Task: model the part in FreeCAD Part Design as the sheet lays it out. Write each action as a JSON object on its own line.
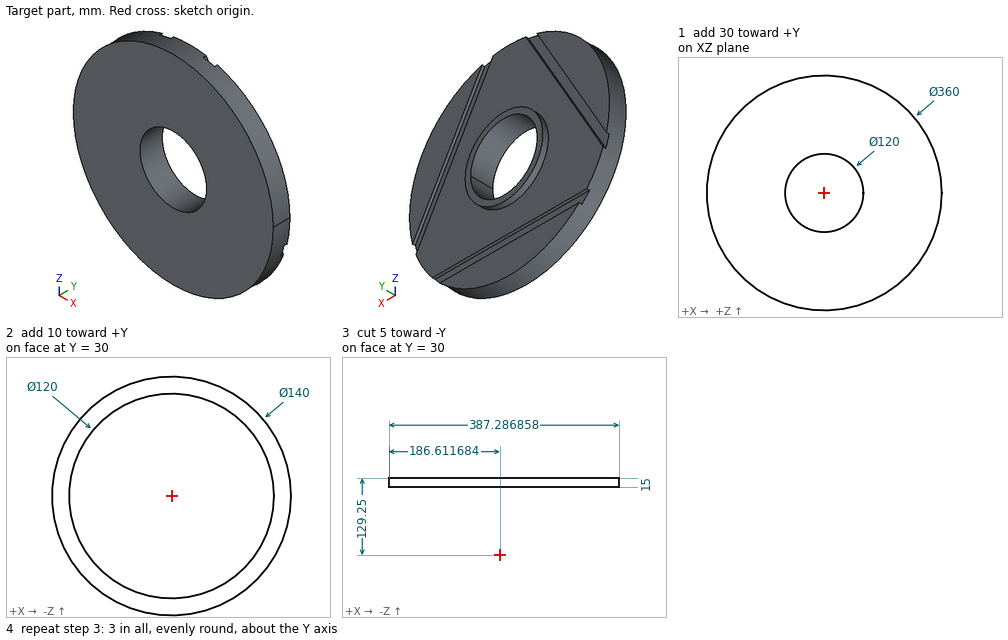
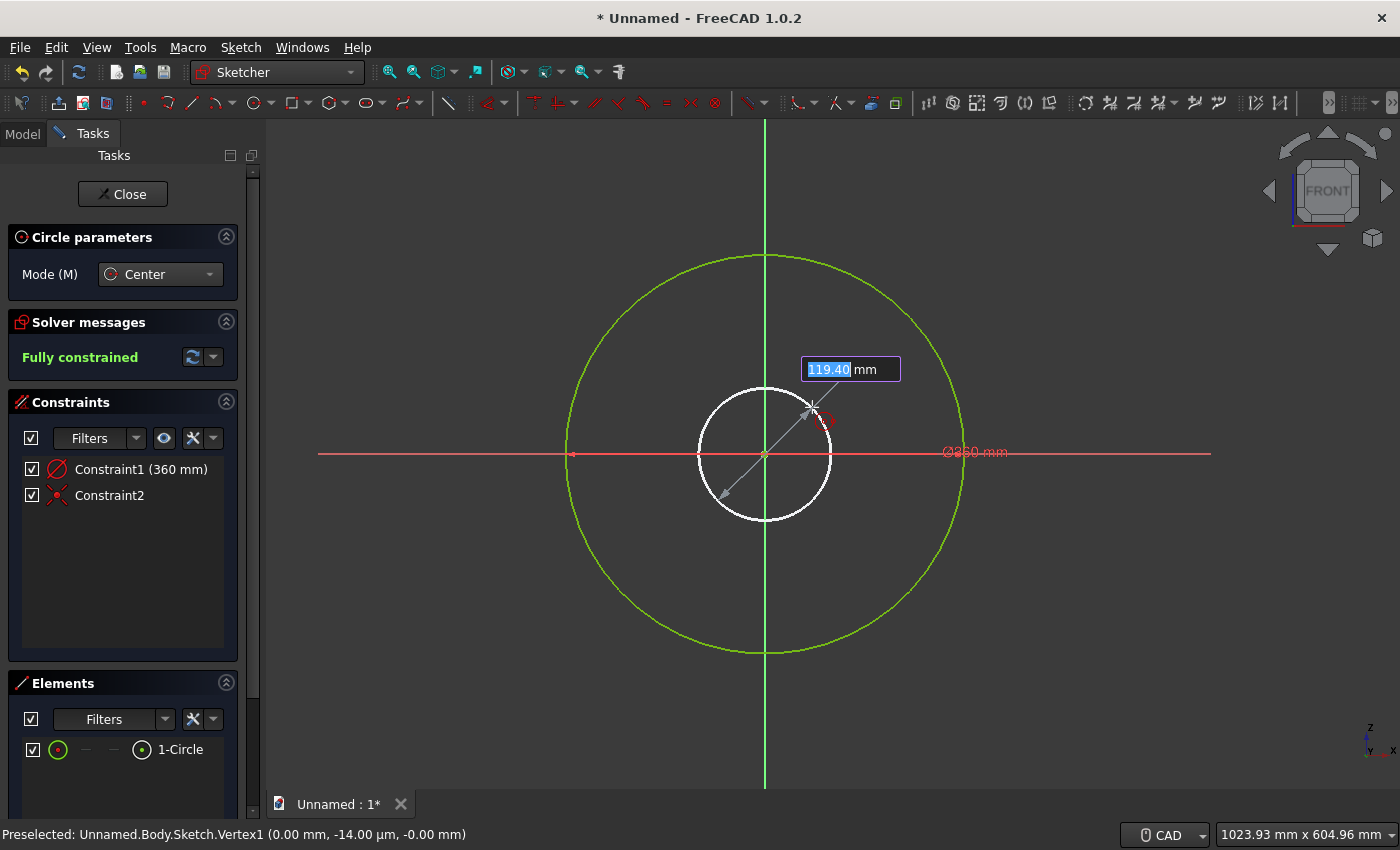
{"action": "type", "text": "120"}
{"action": "key", "text": "Return"}
{"action": "key", "text": "Escape"}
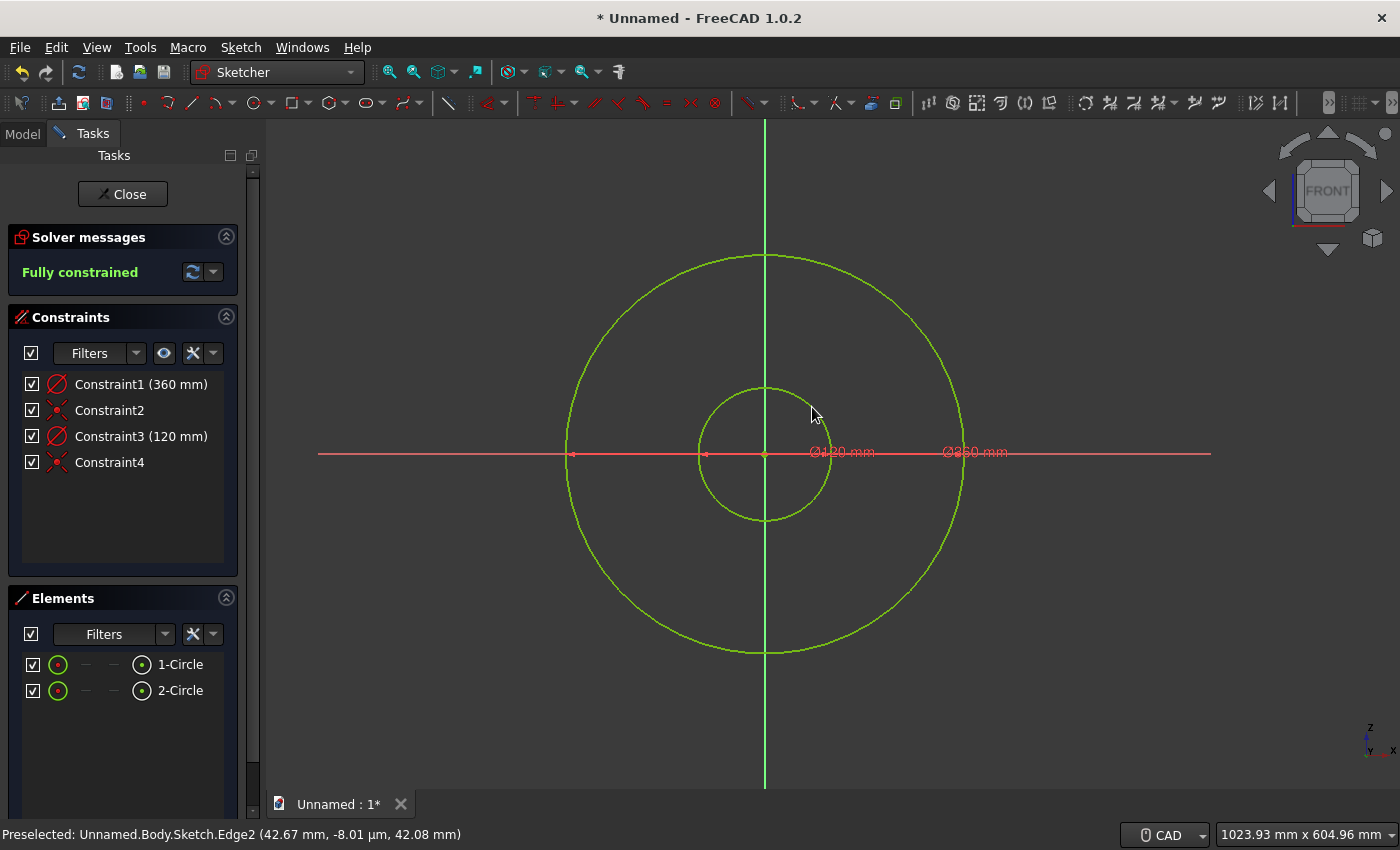
{"action": "left_click", "coordinate": [123, 194]}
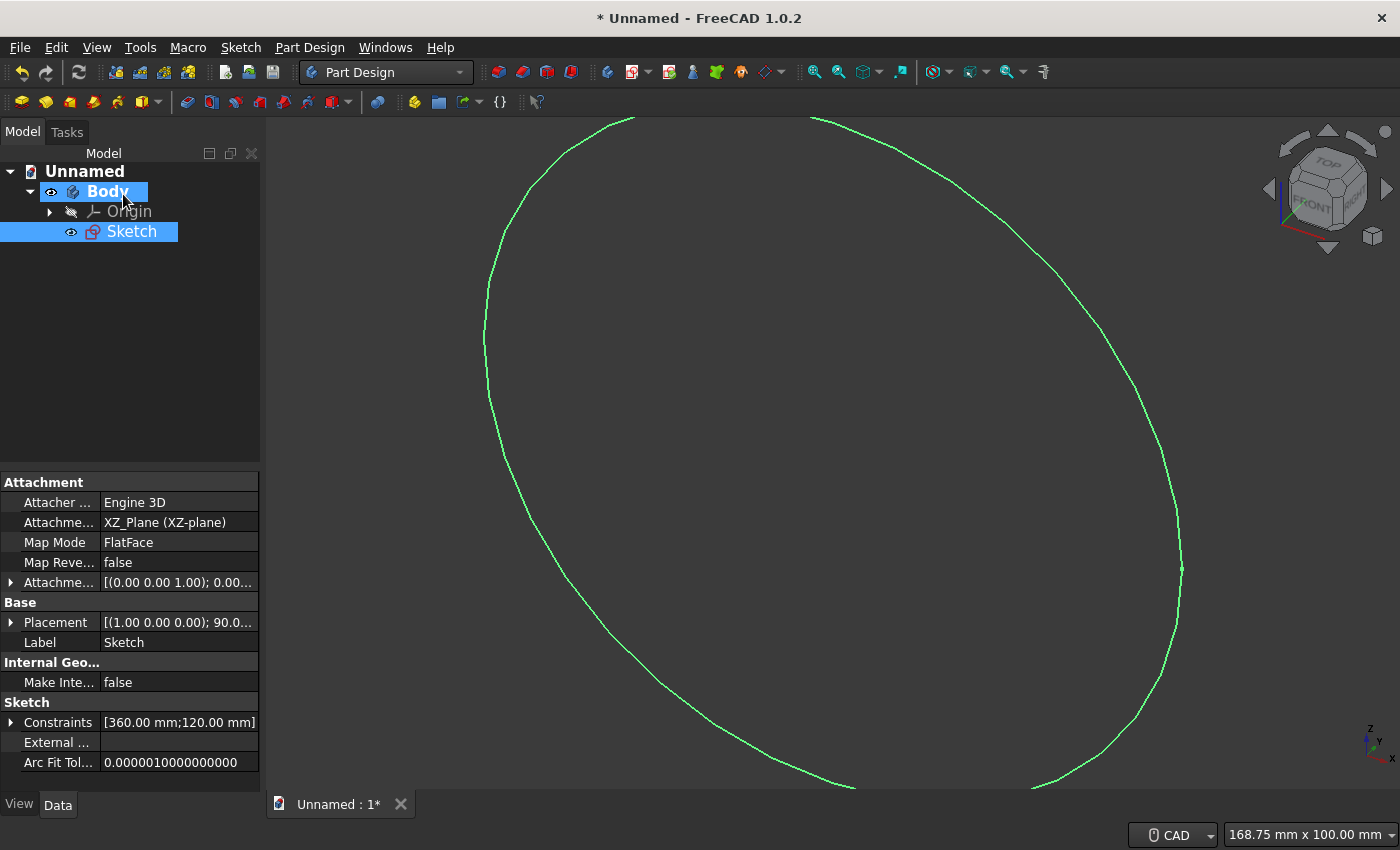
{"action": "left_click", "coordinate": [22, 102]}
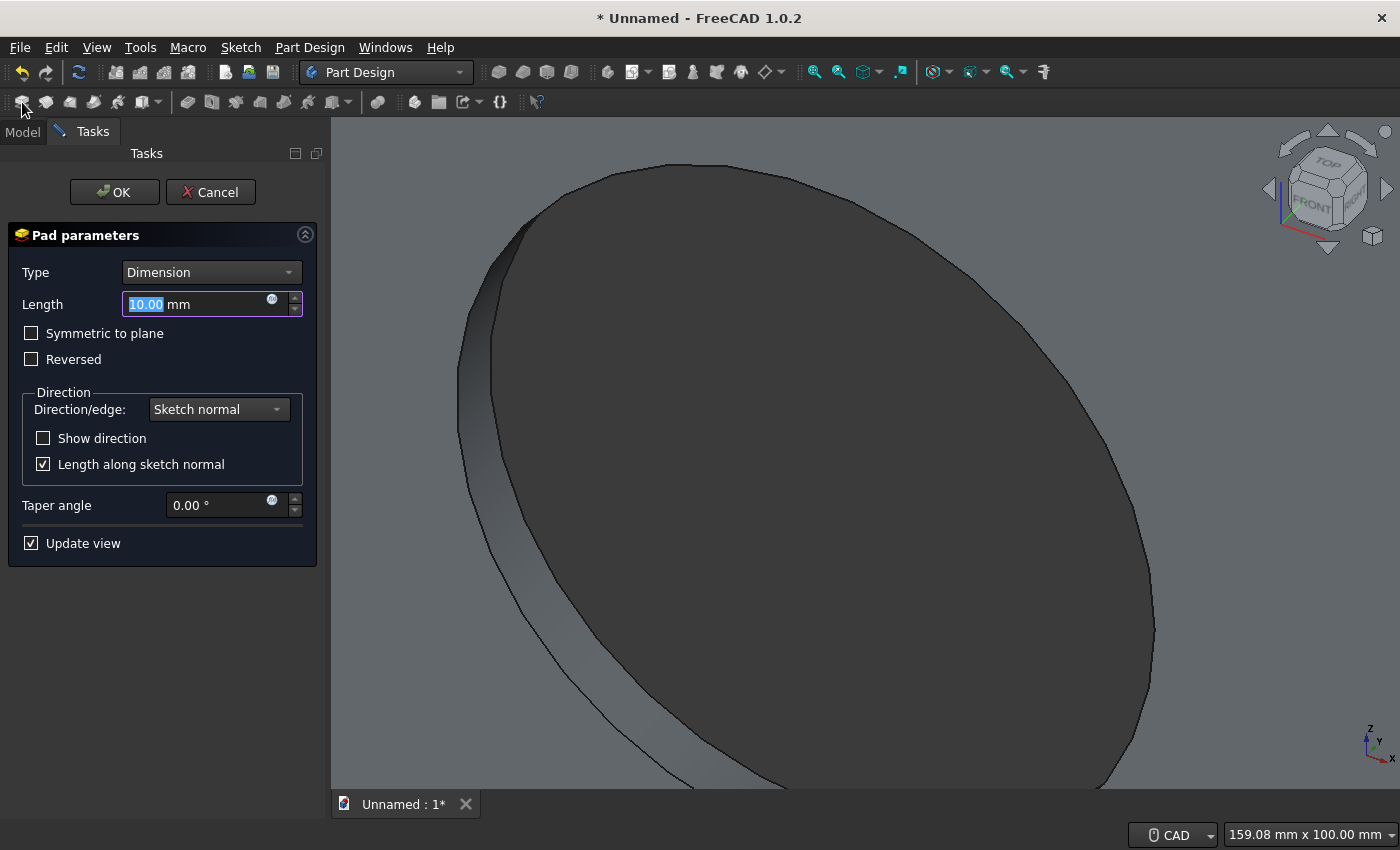
{"action": "type", "text": "30"}
{"action": "key", "text": "Tab"}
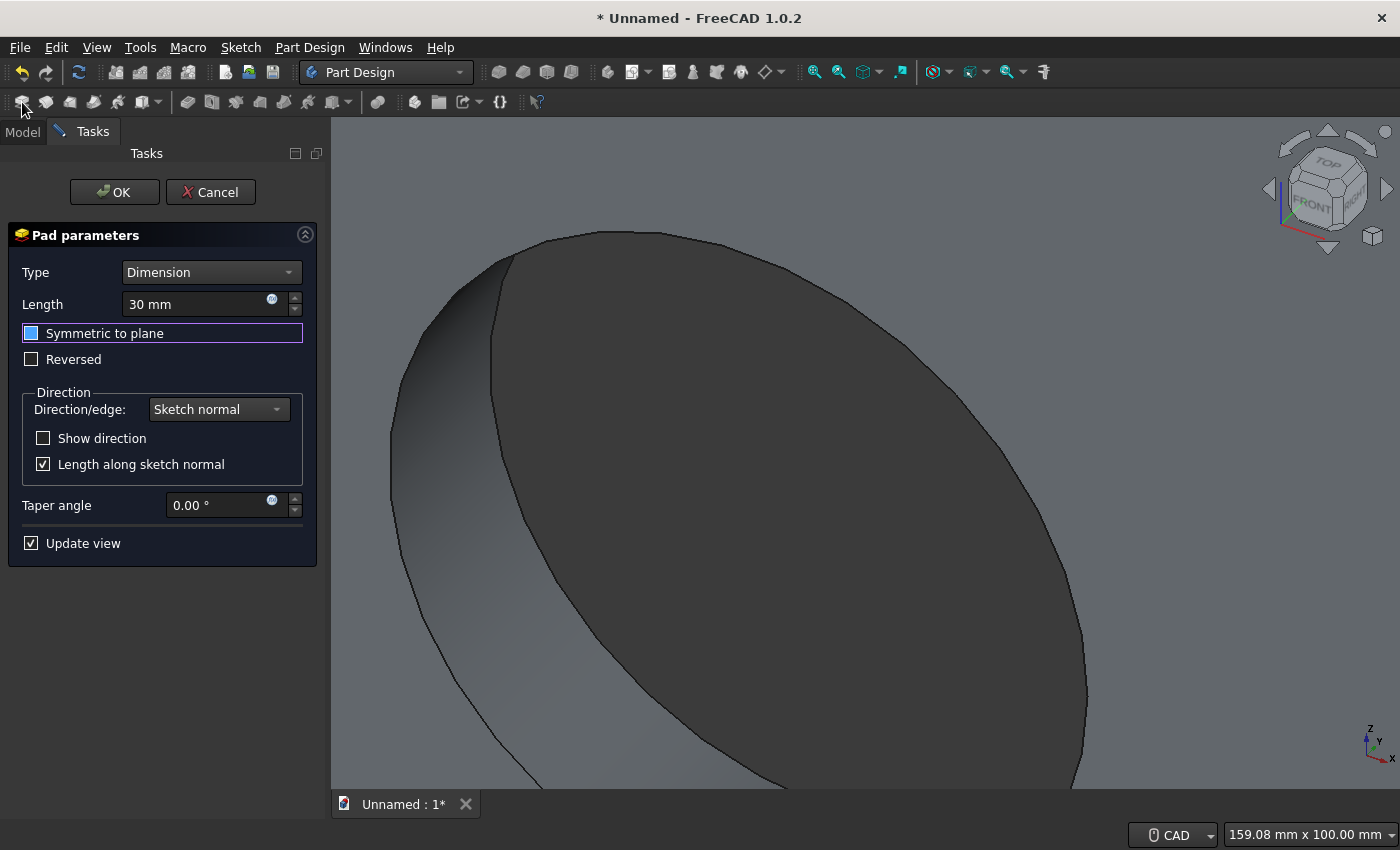
{"action": "left_click", "coordinate": [30, 359]}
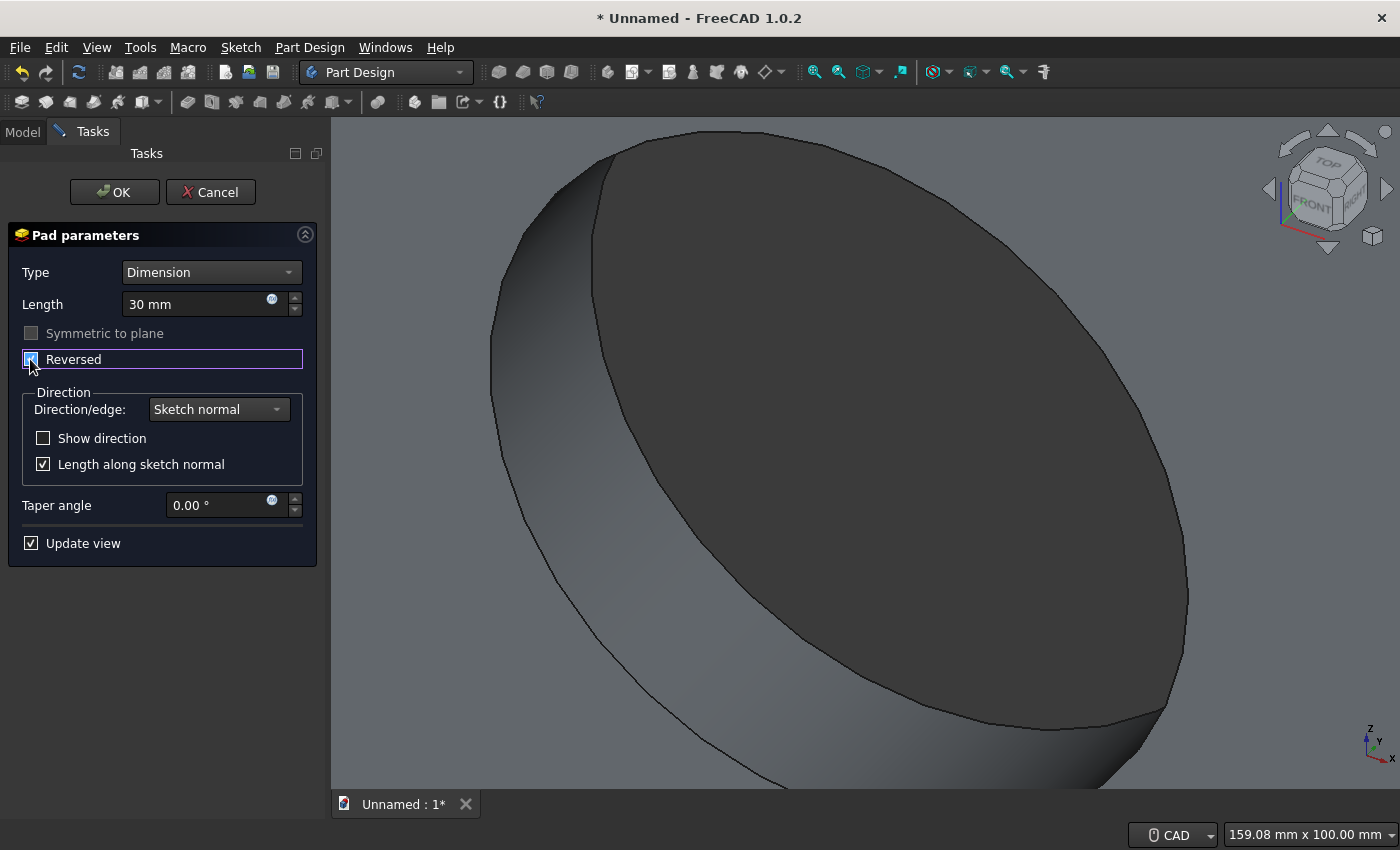
{"action": "left_click", "coordinate": [115, 192]}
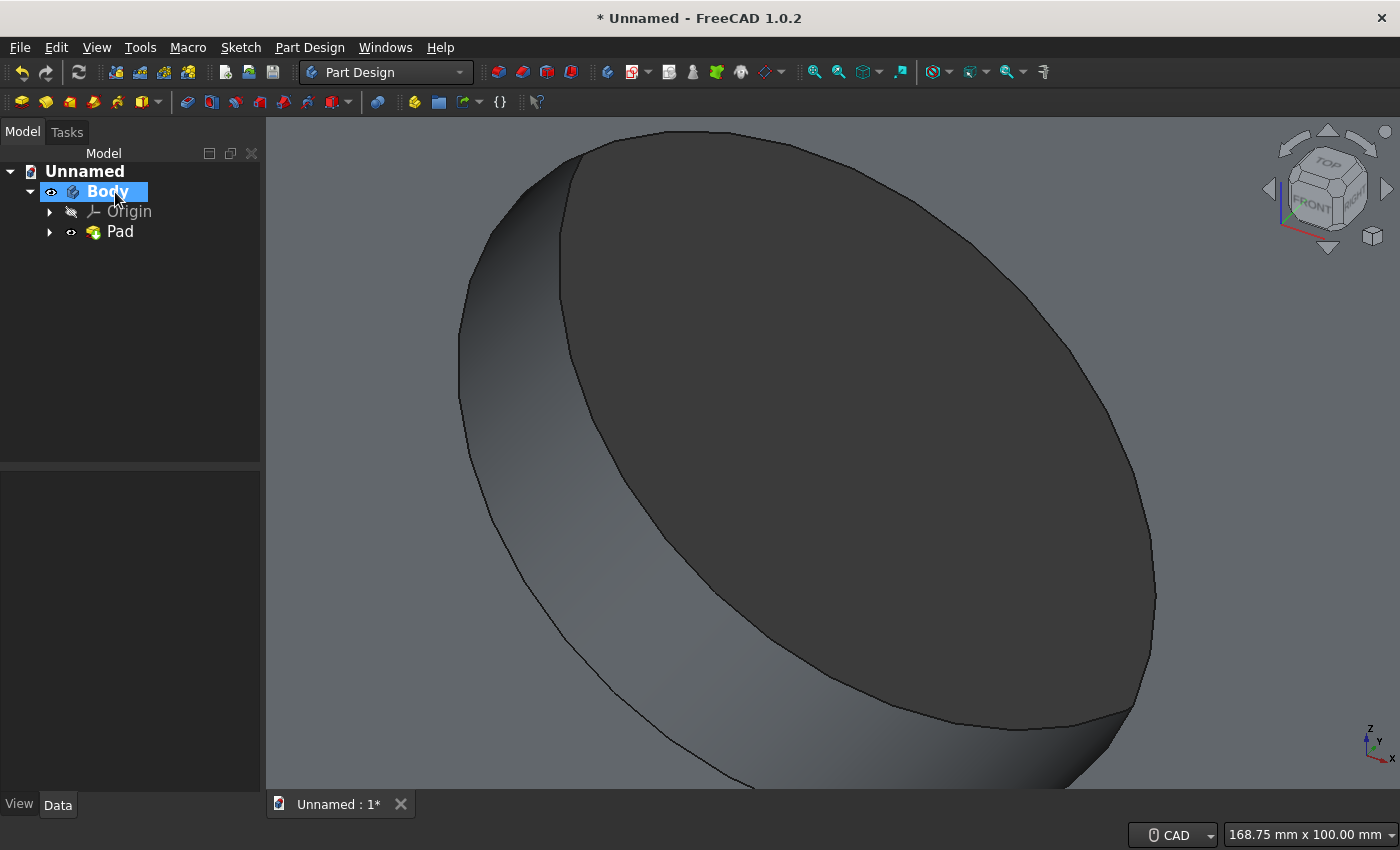
{"action": "left_click", "coordinate": [816, 72]}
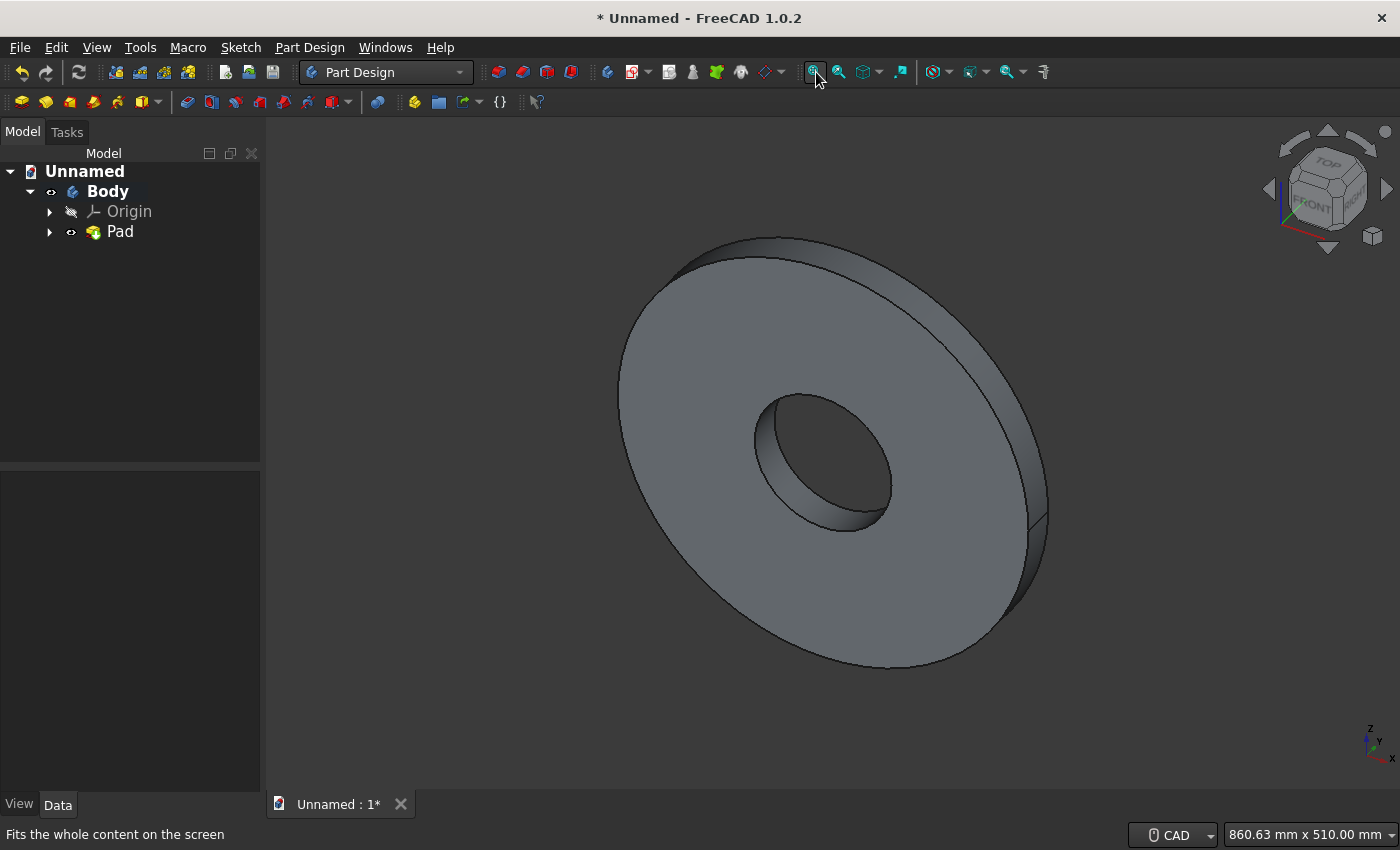
{"action": "key", "text": "4"}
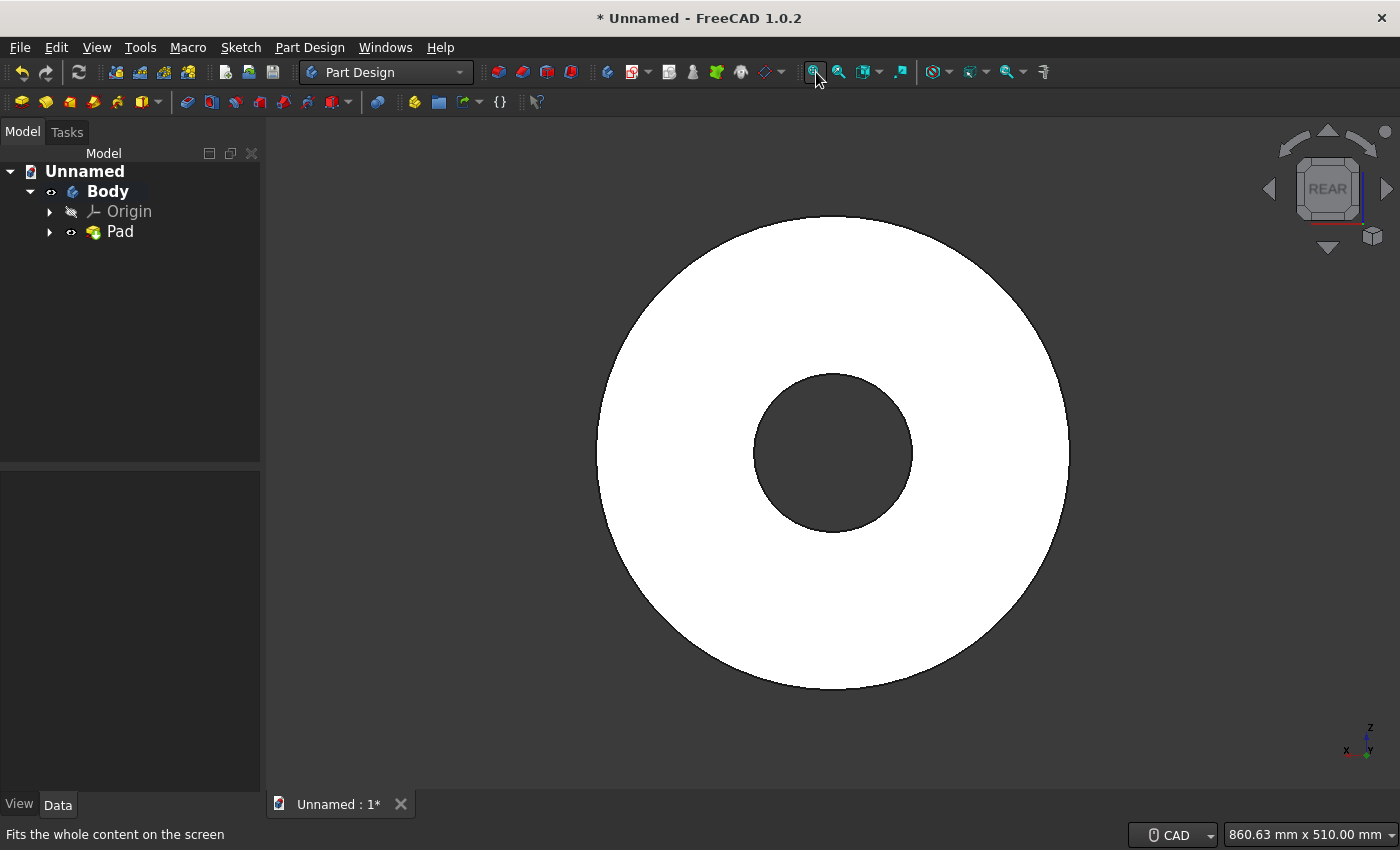
{"action": "left_click", "coordinate": [901, 588]}